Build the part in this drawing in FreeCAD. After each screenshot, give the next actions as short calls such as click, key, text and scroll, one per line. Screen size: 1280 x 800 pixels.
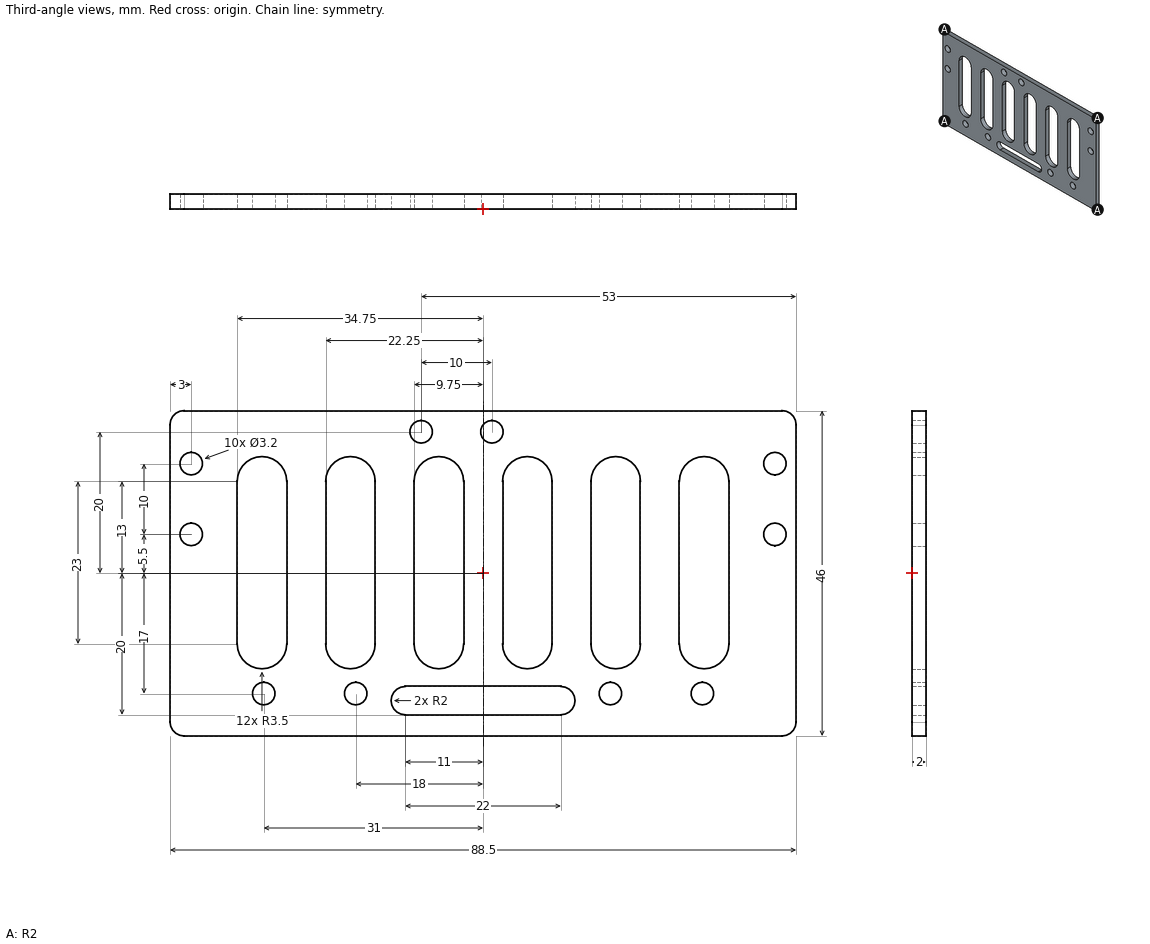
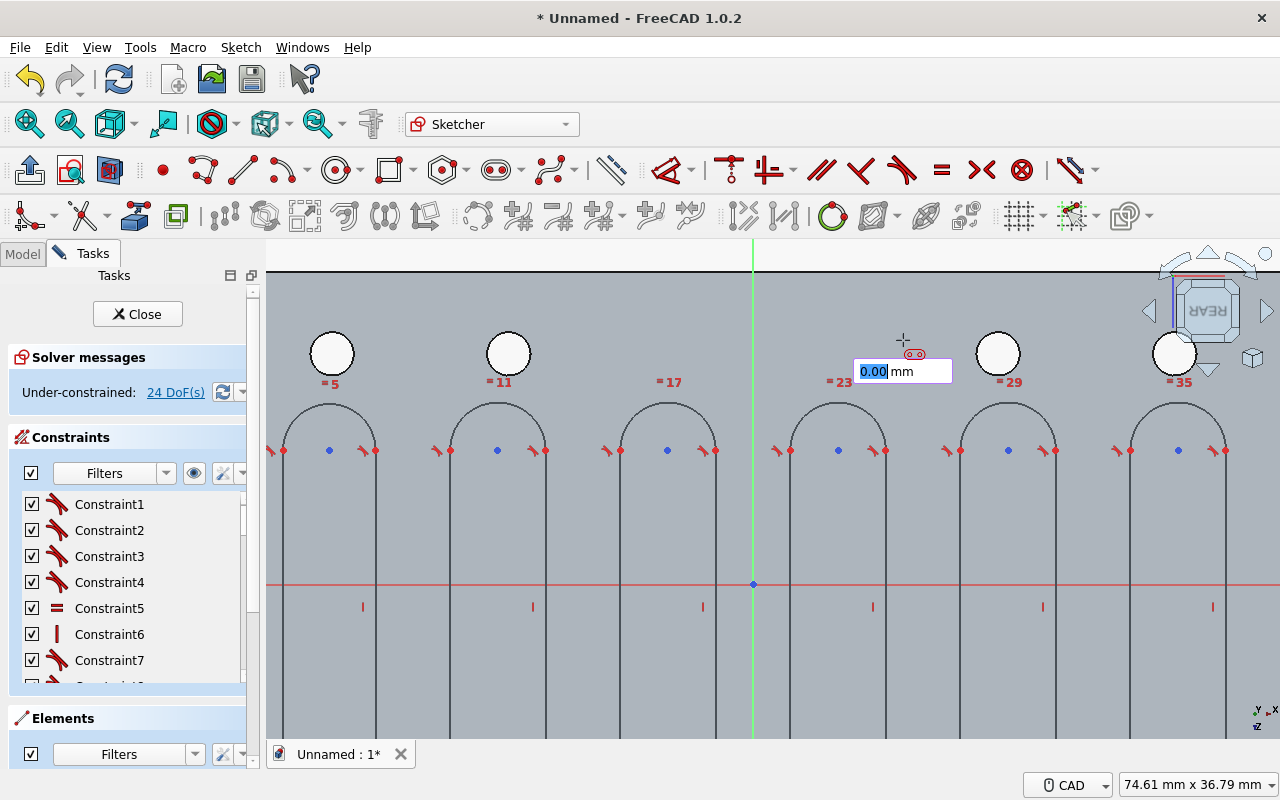
click(798, 313)
key(Escape)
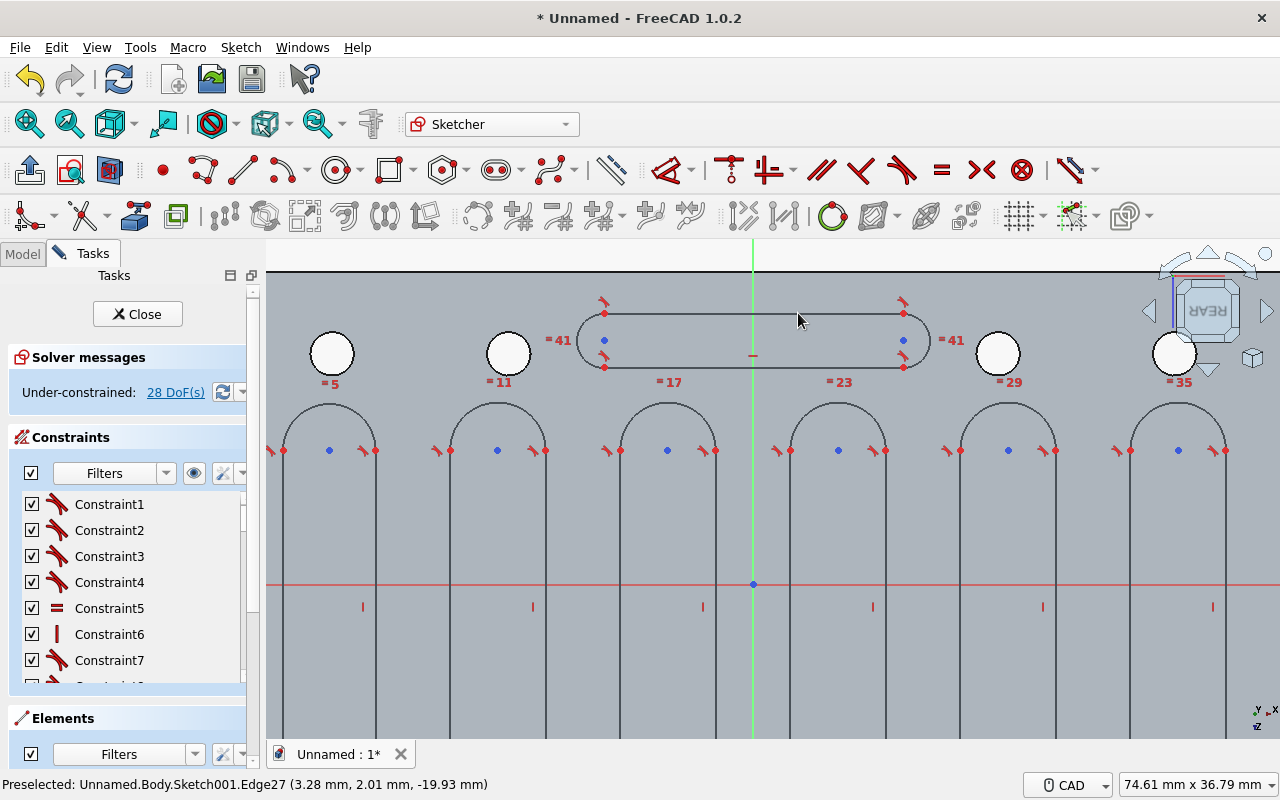
scroll(605, 342, down, 2)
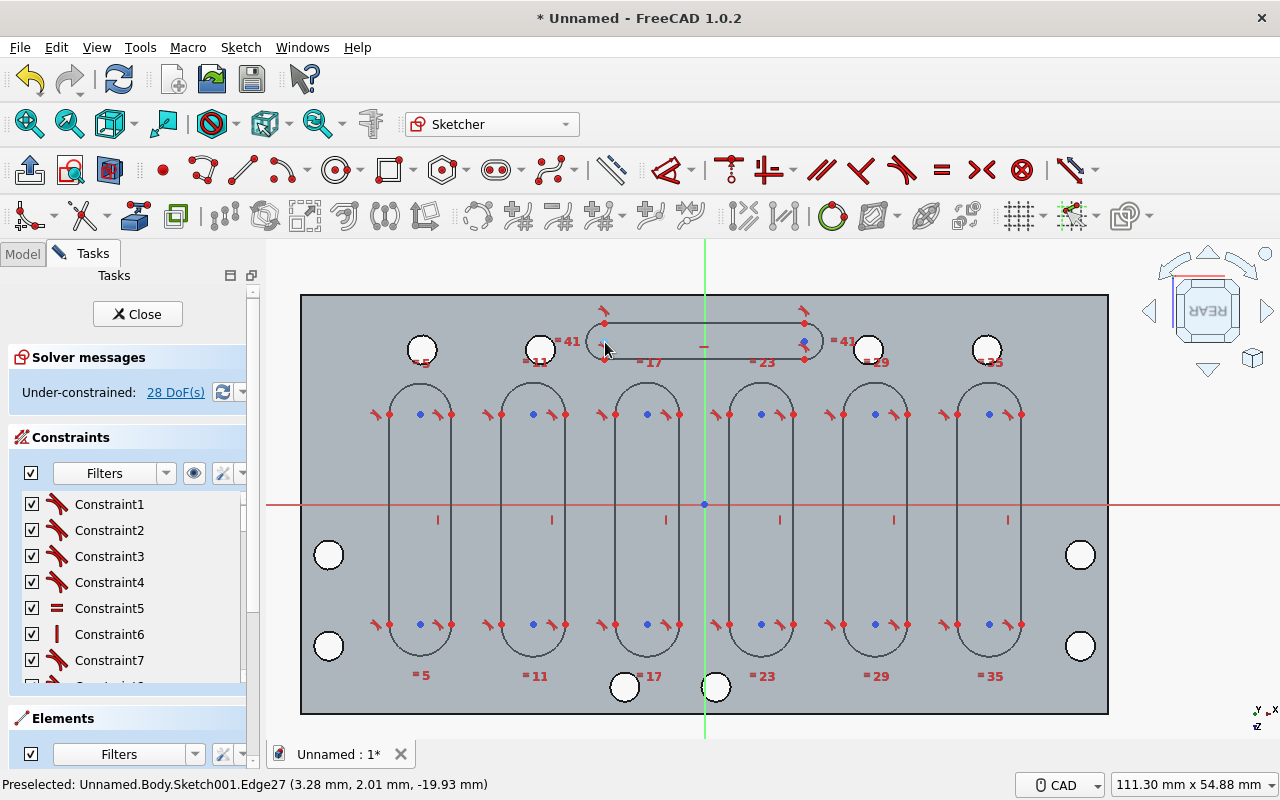
click(402, 650)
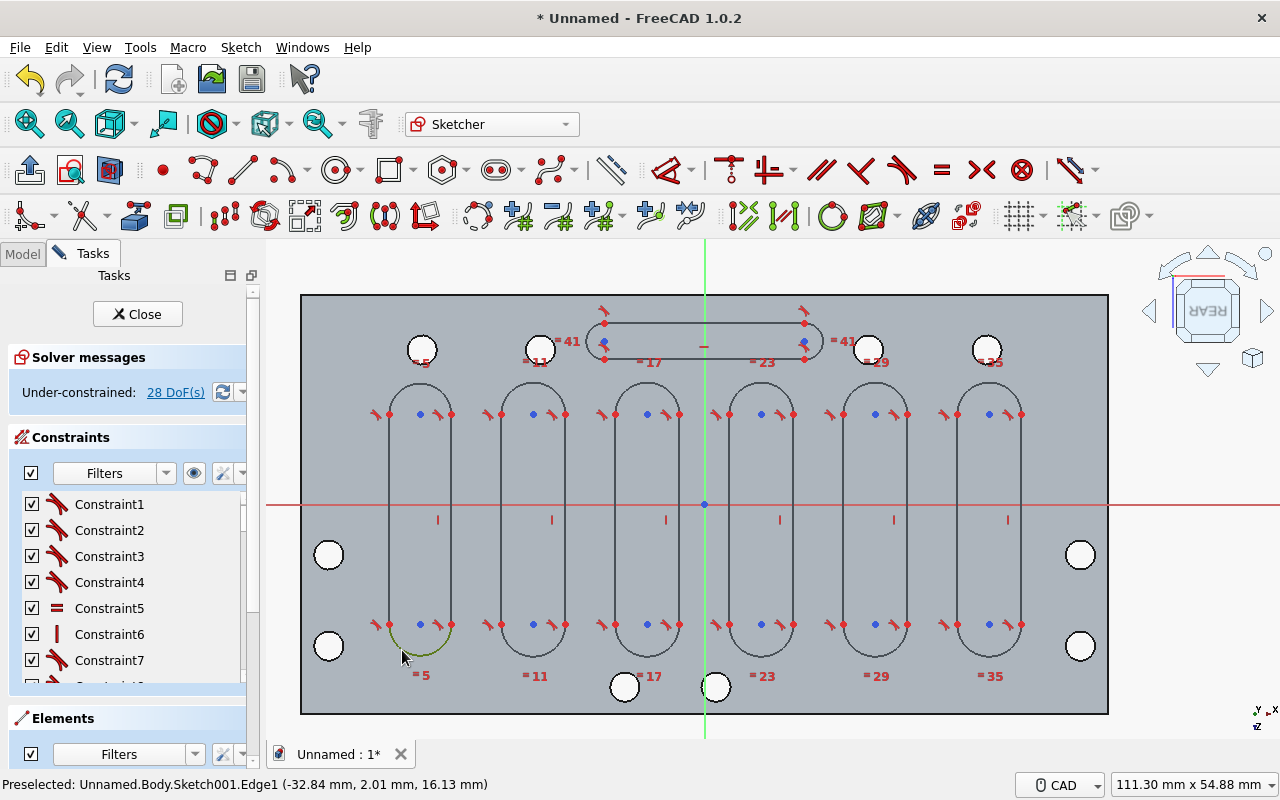
click(515, 651)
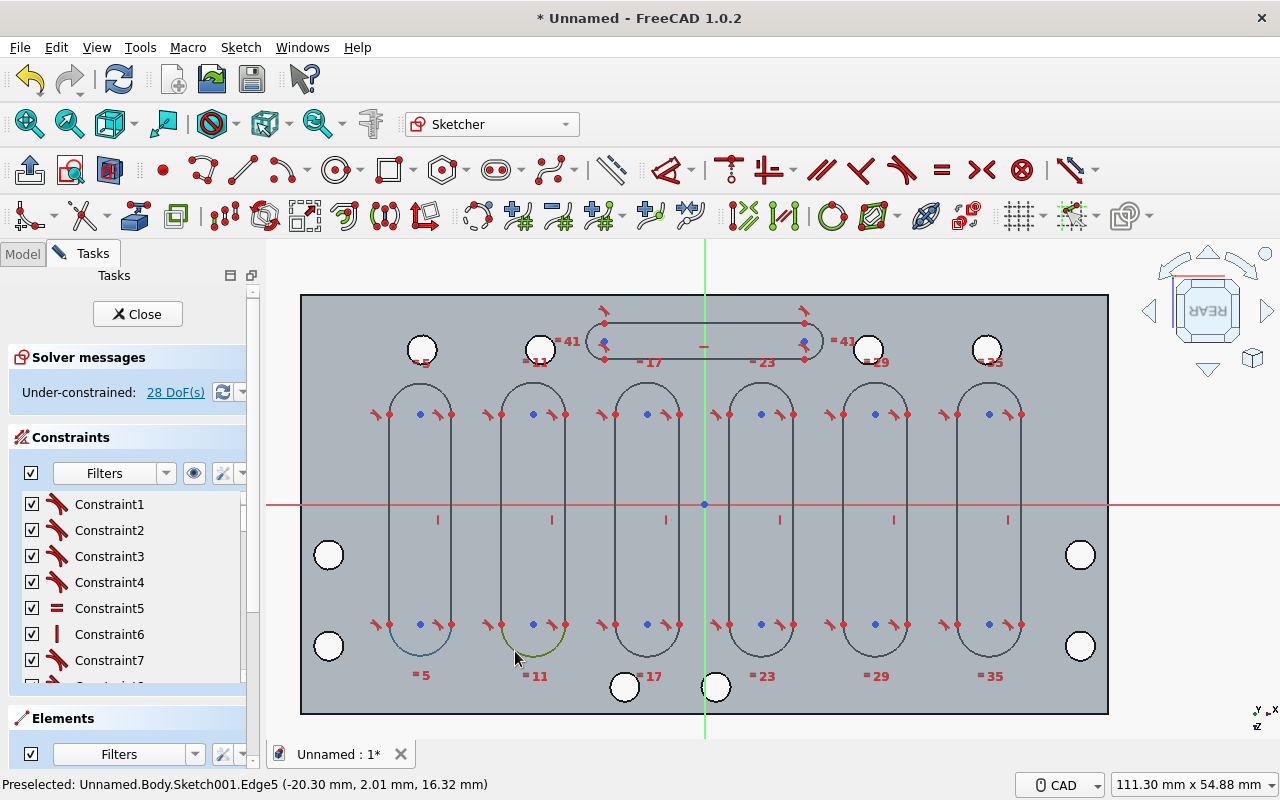
click(629, 651)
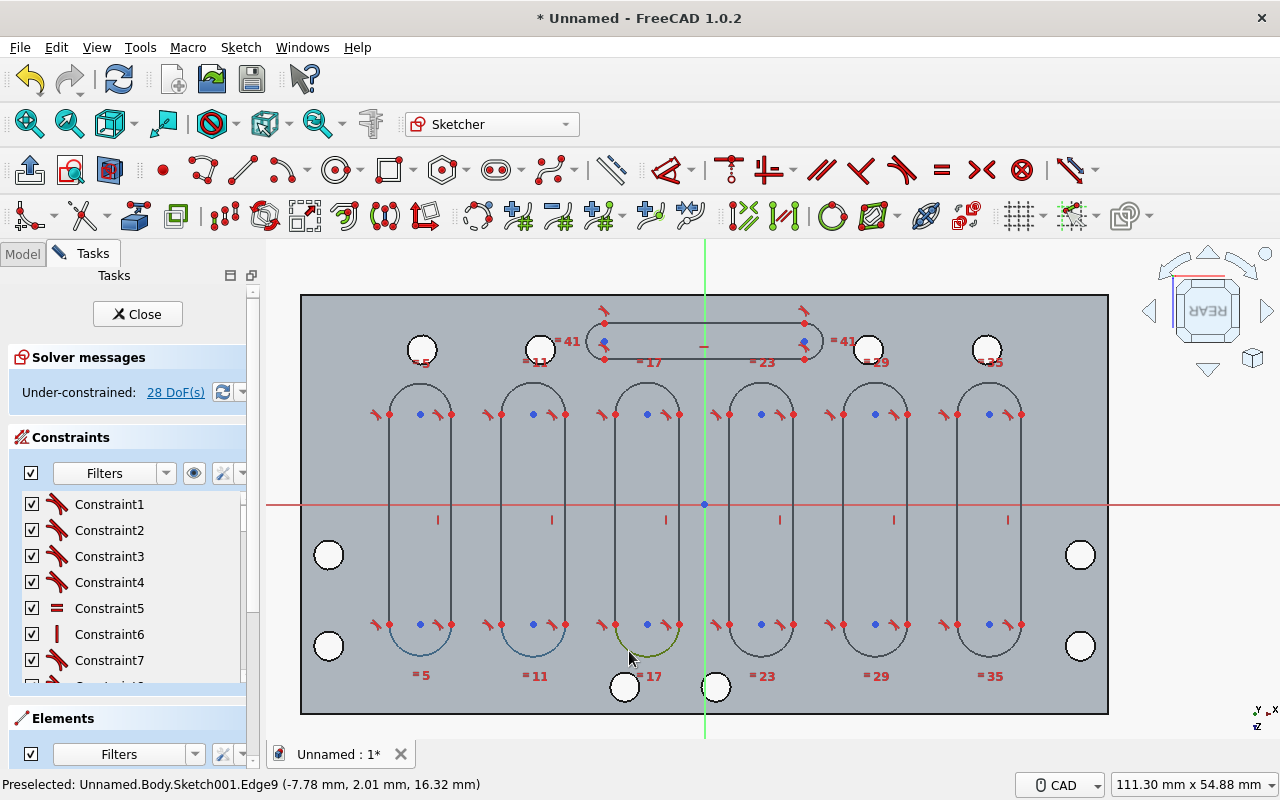
click(743, 651)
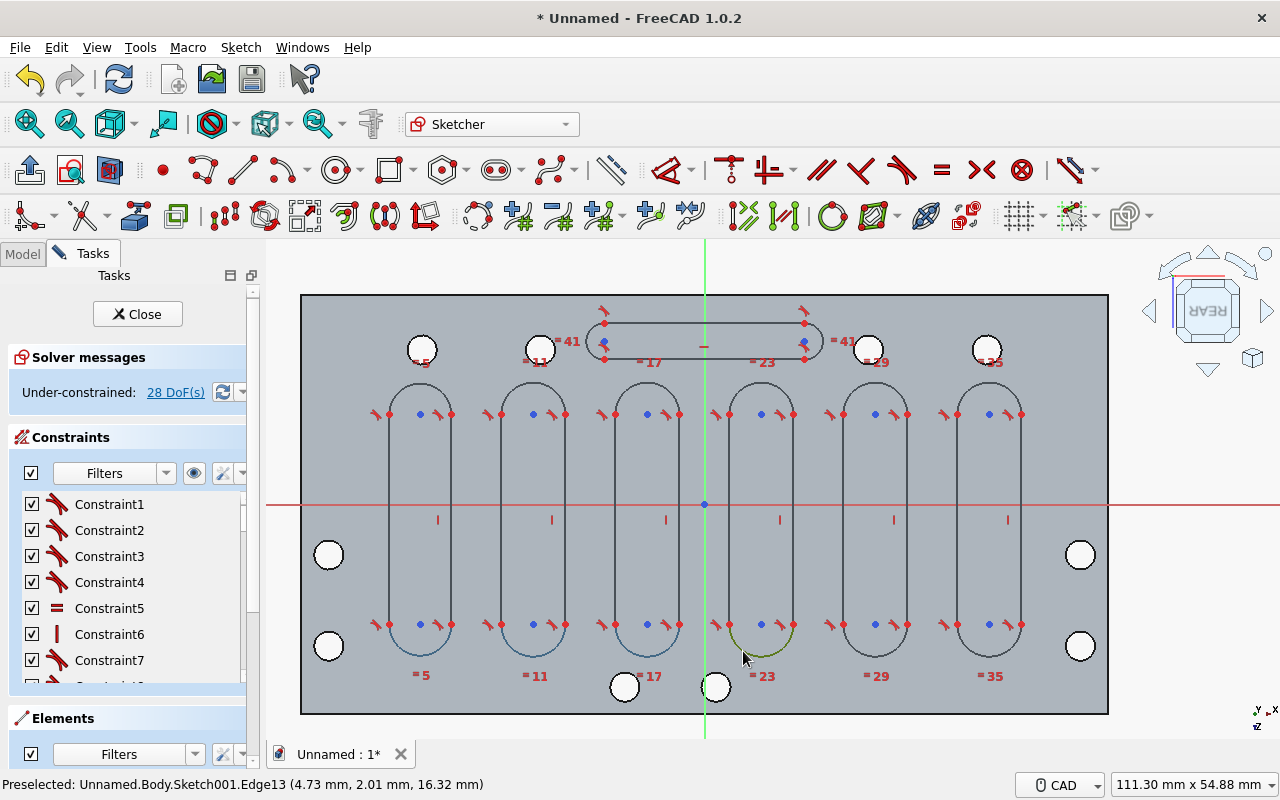
click(857, 651)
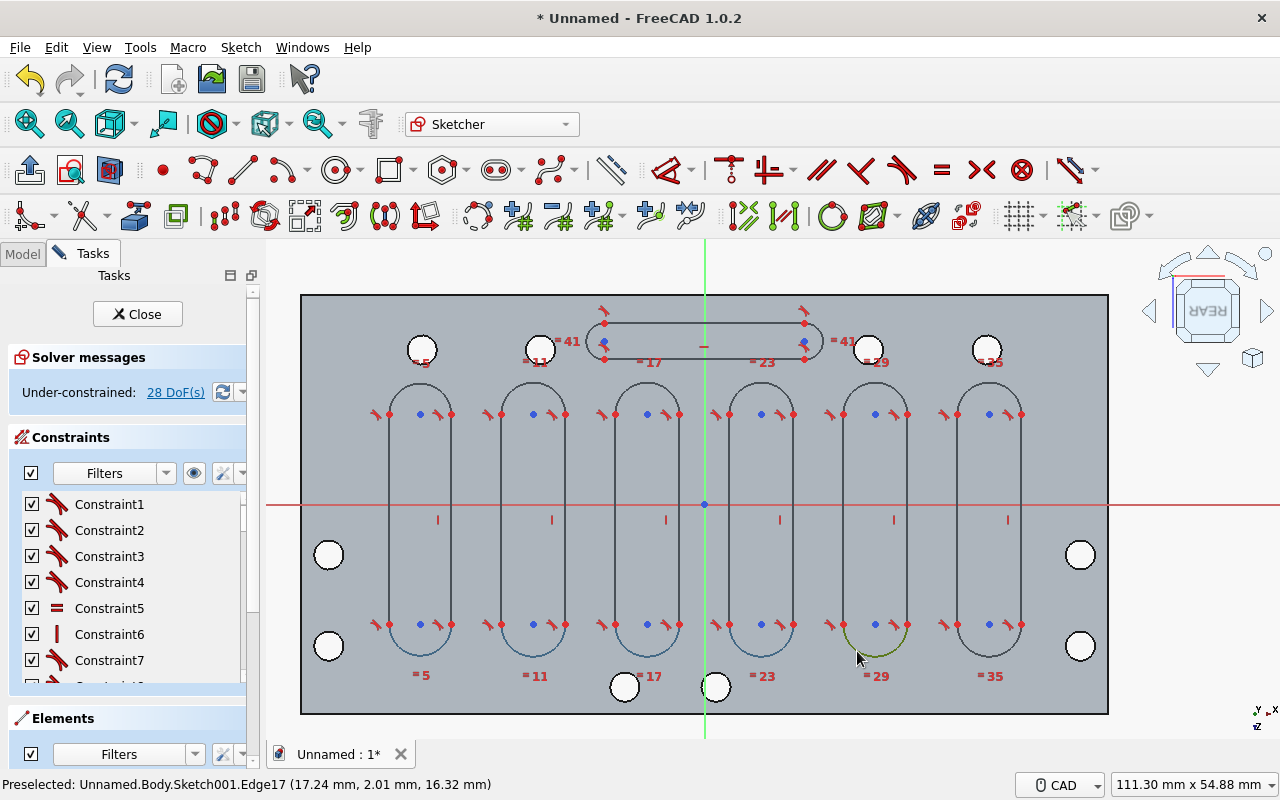
click(971, 651)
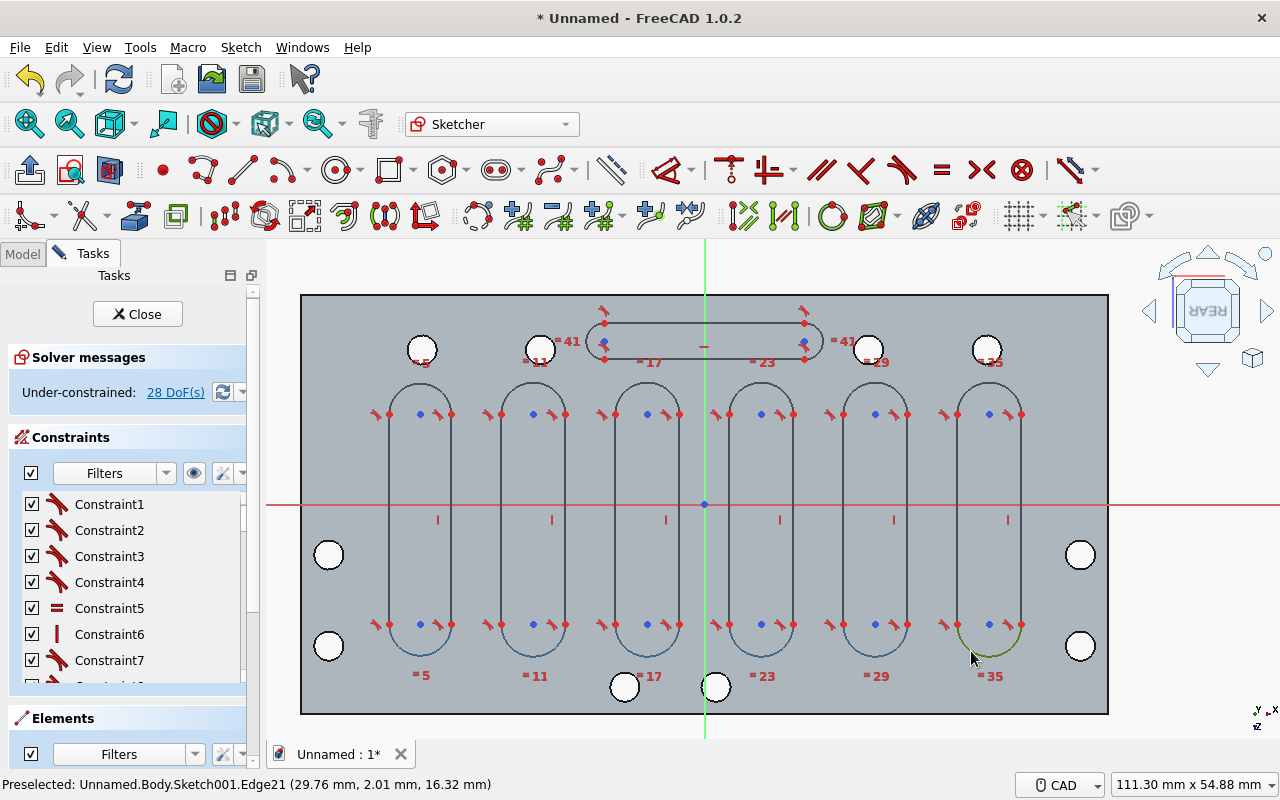
click(942, 170)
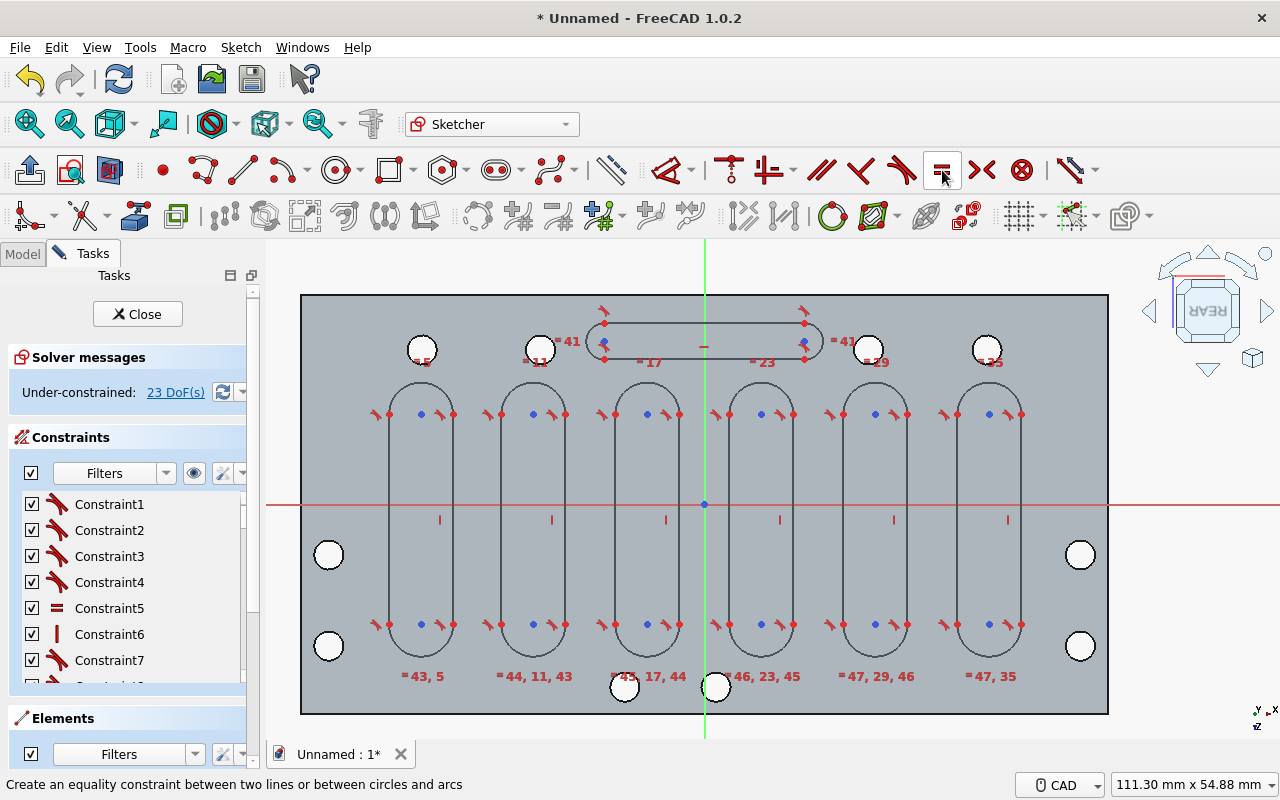
click(647, 625)